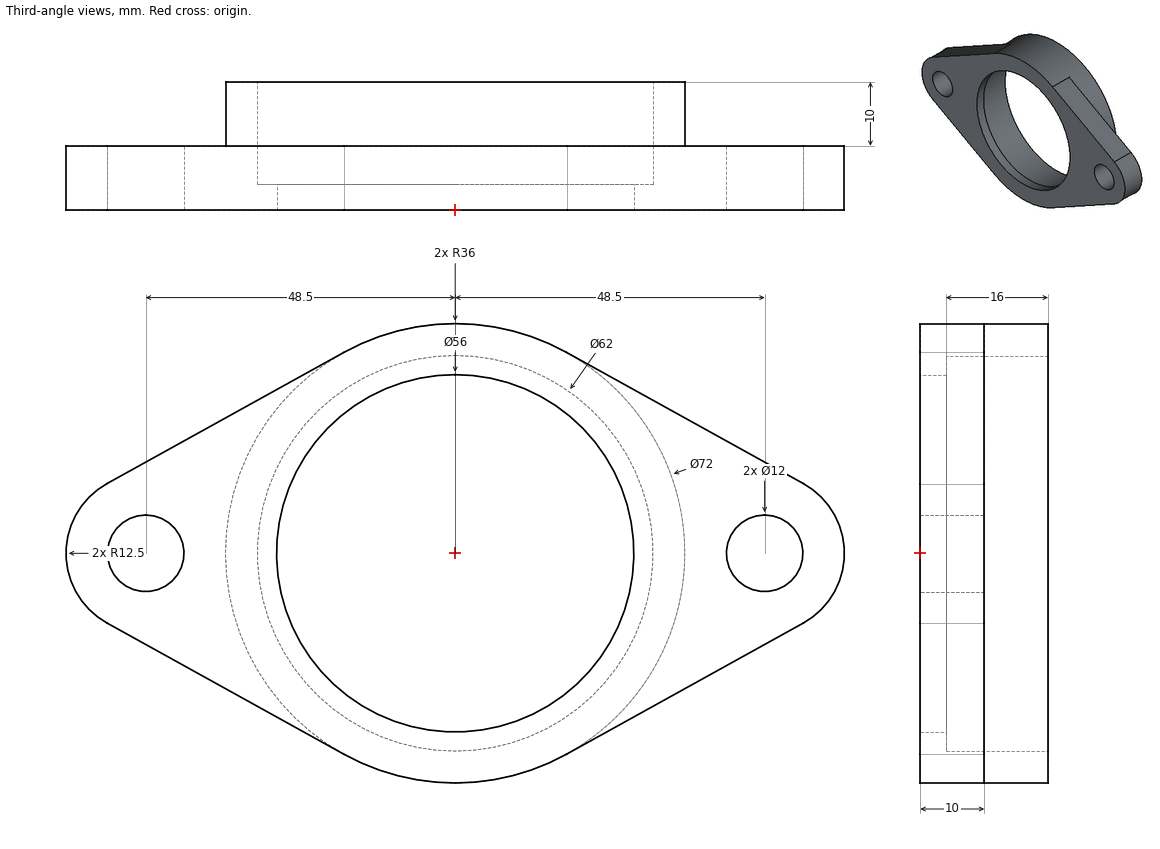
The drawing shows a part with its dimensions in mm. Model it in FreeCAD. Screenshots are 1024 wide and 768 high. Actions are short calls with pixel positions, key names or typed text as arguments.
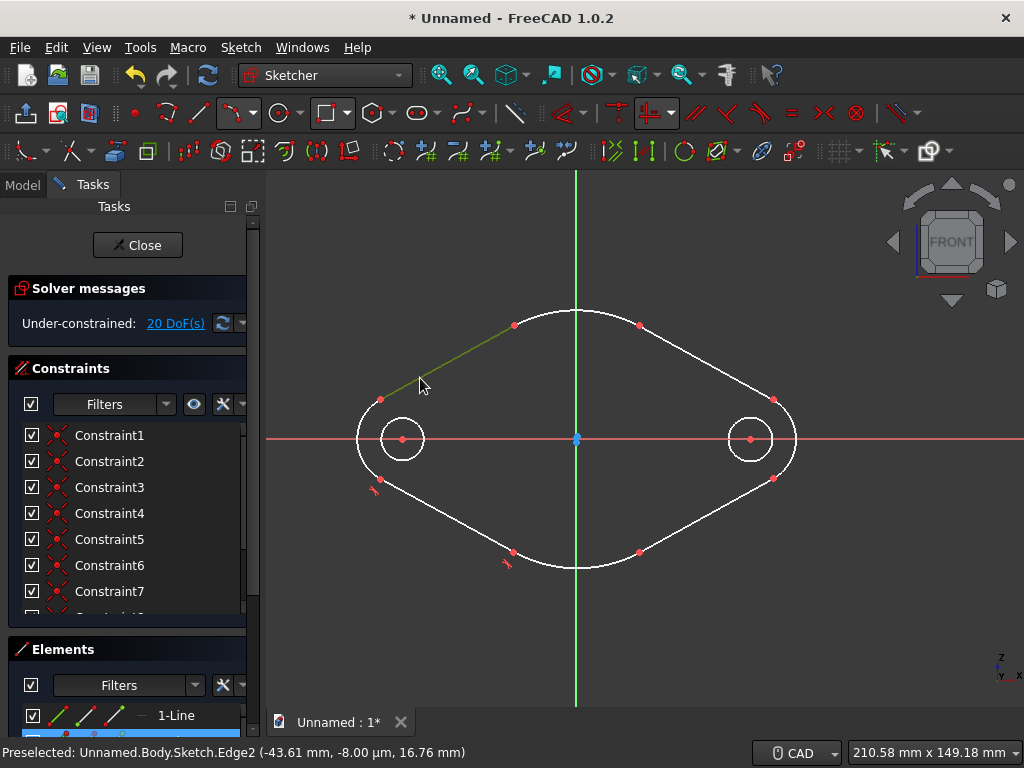
click(361, 421)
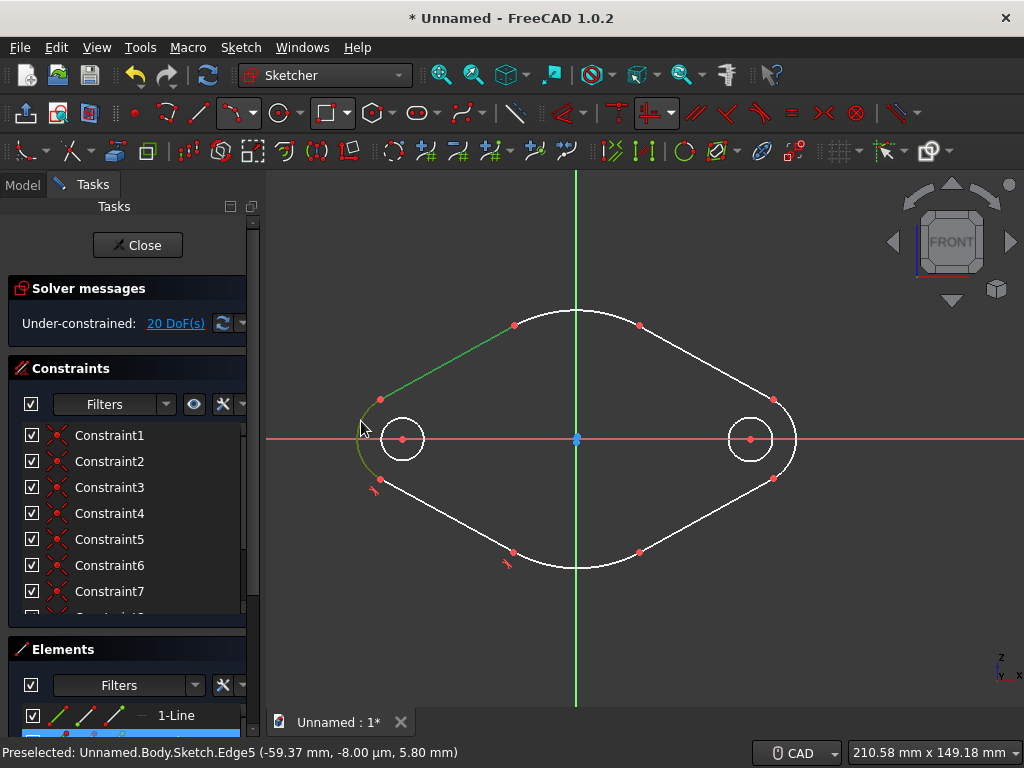
click(760, 114)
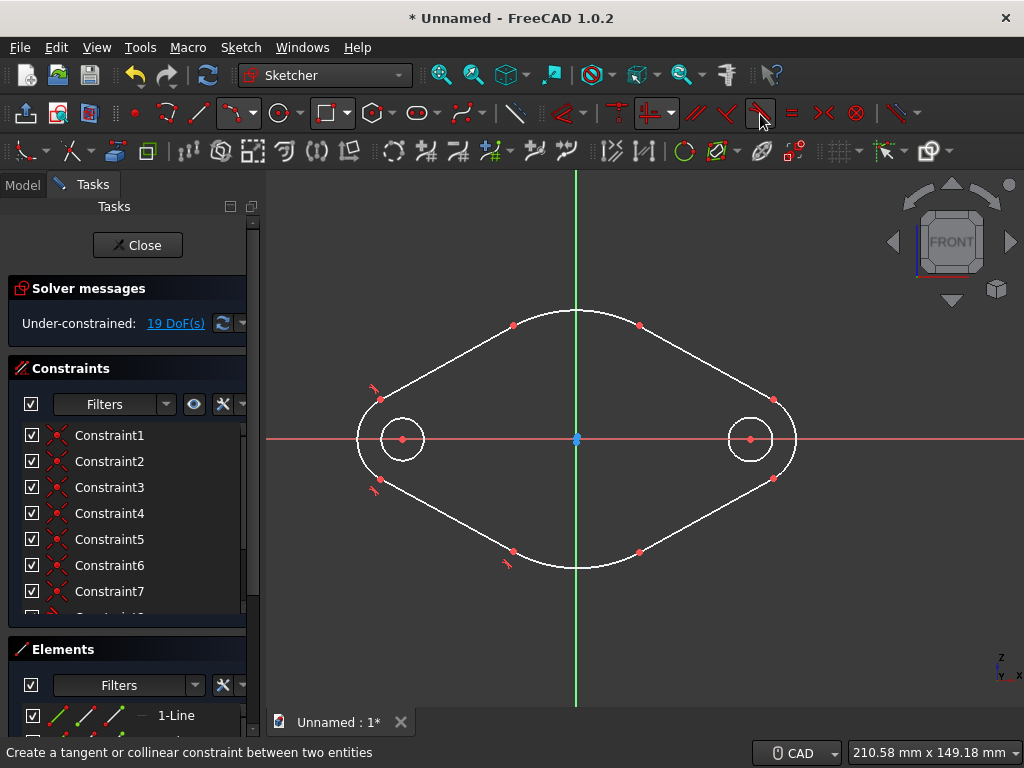
click(421, 378)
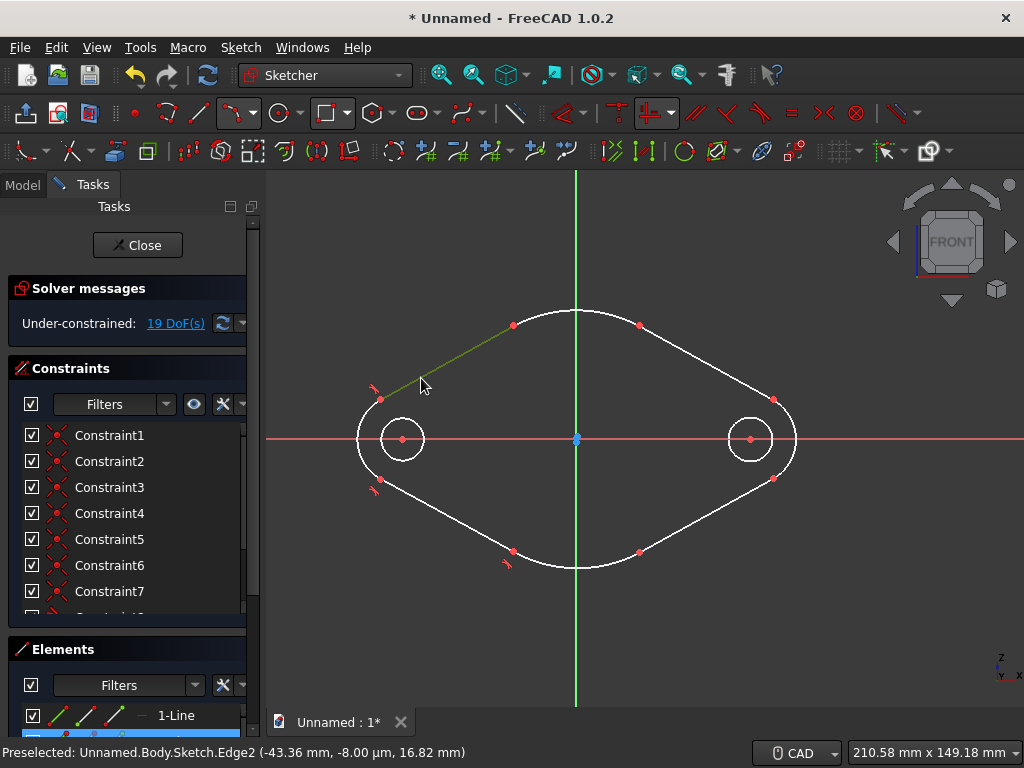
click(602, 313)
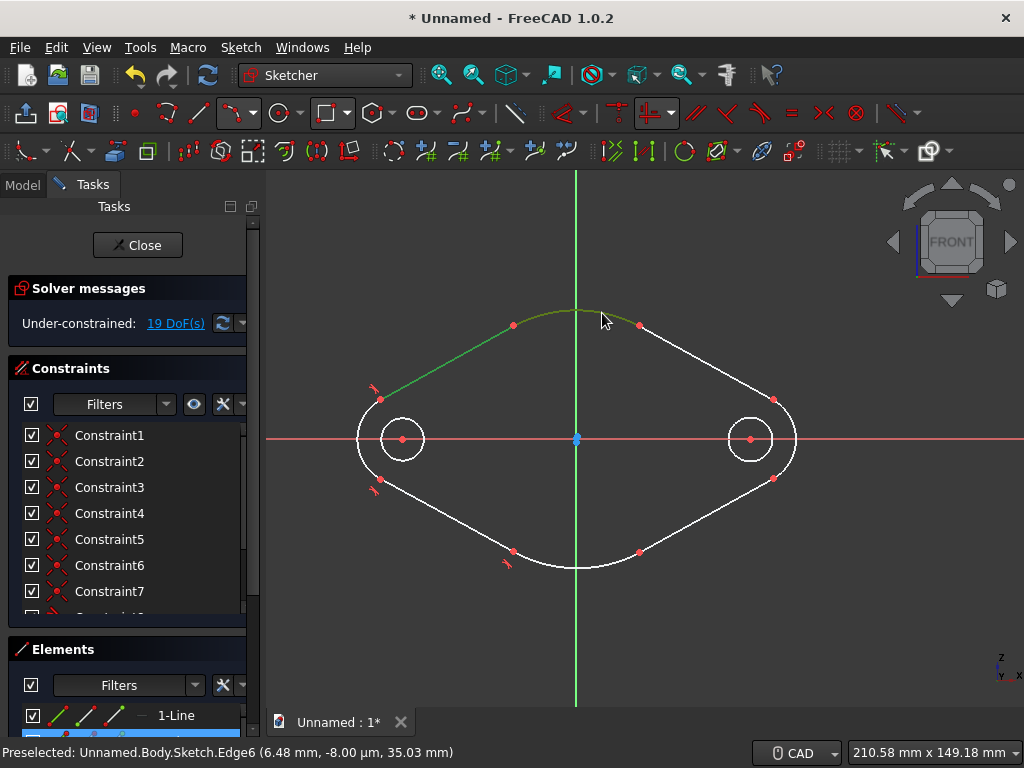
click(760, 114)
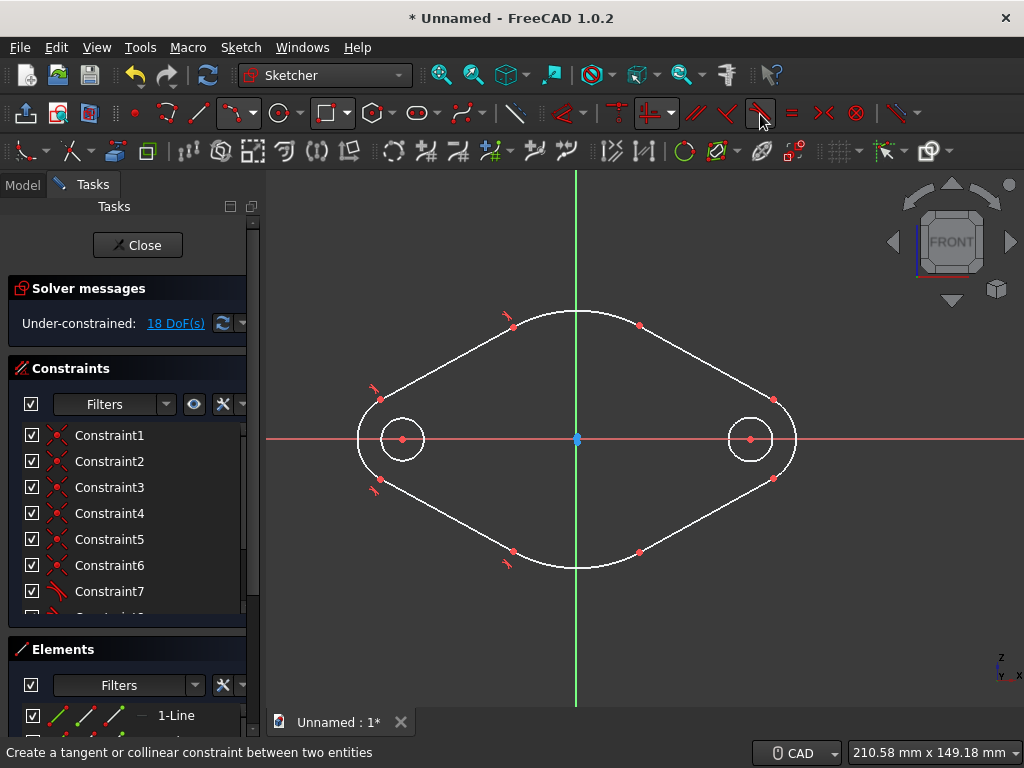
click(679, 348)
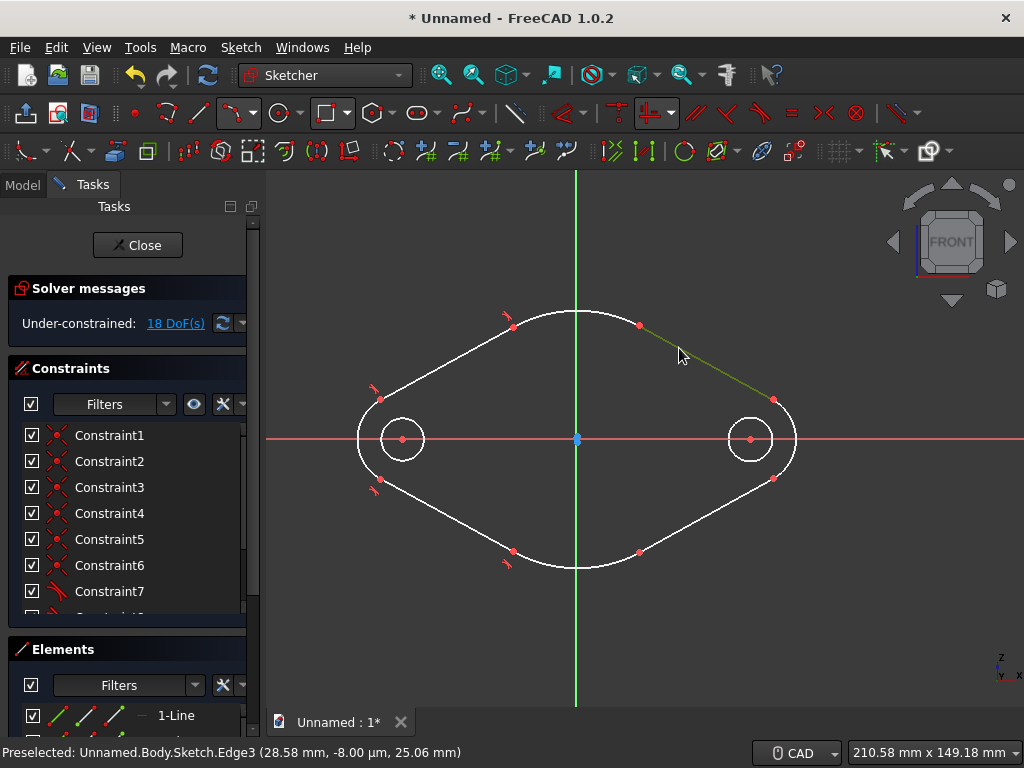
click(602, 313)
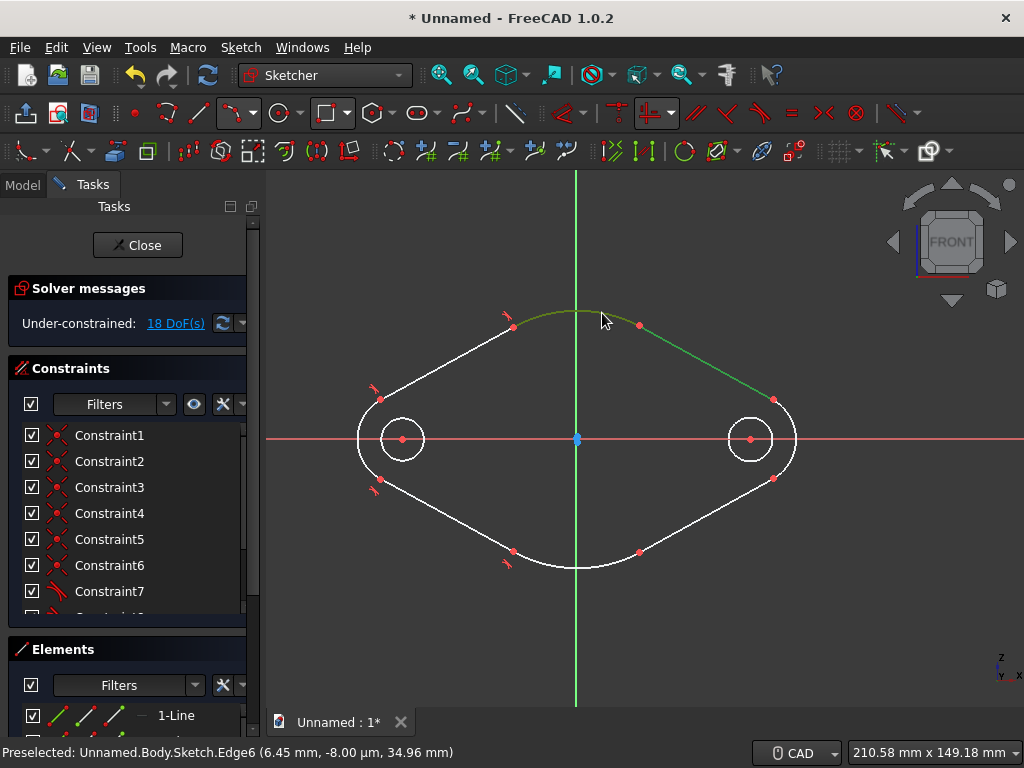
click(760, 114)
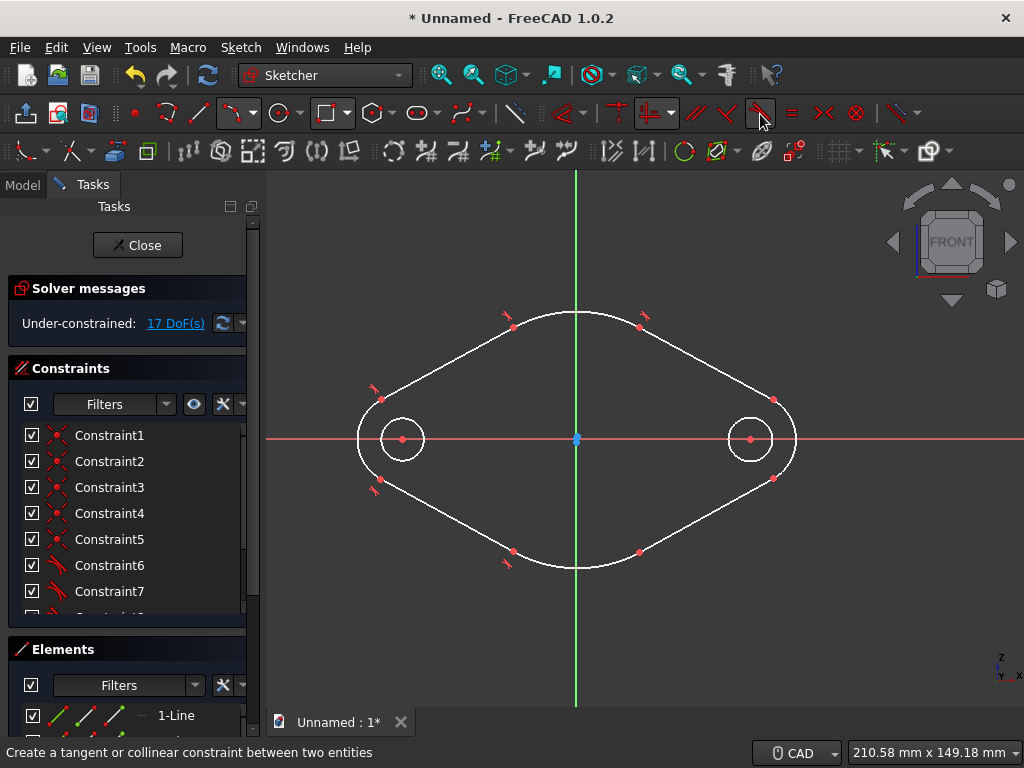
click(679, 349)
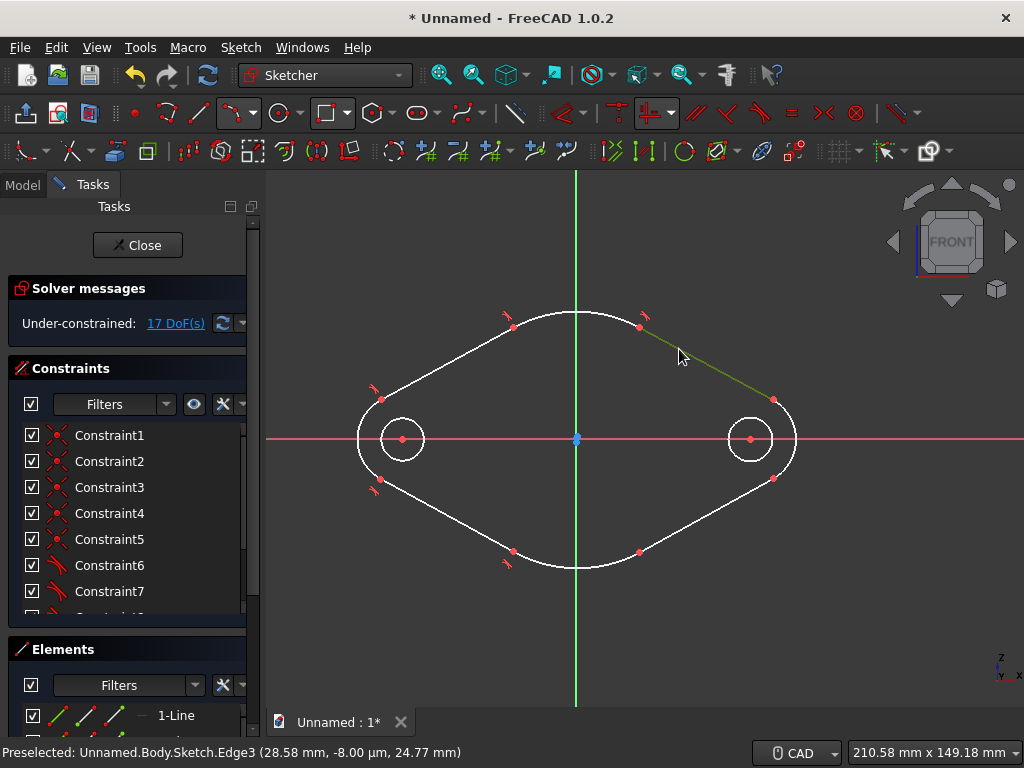
click(792, 458)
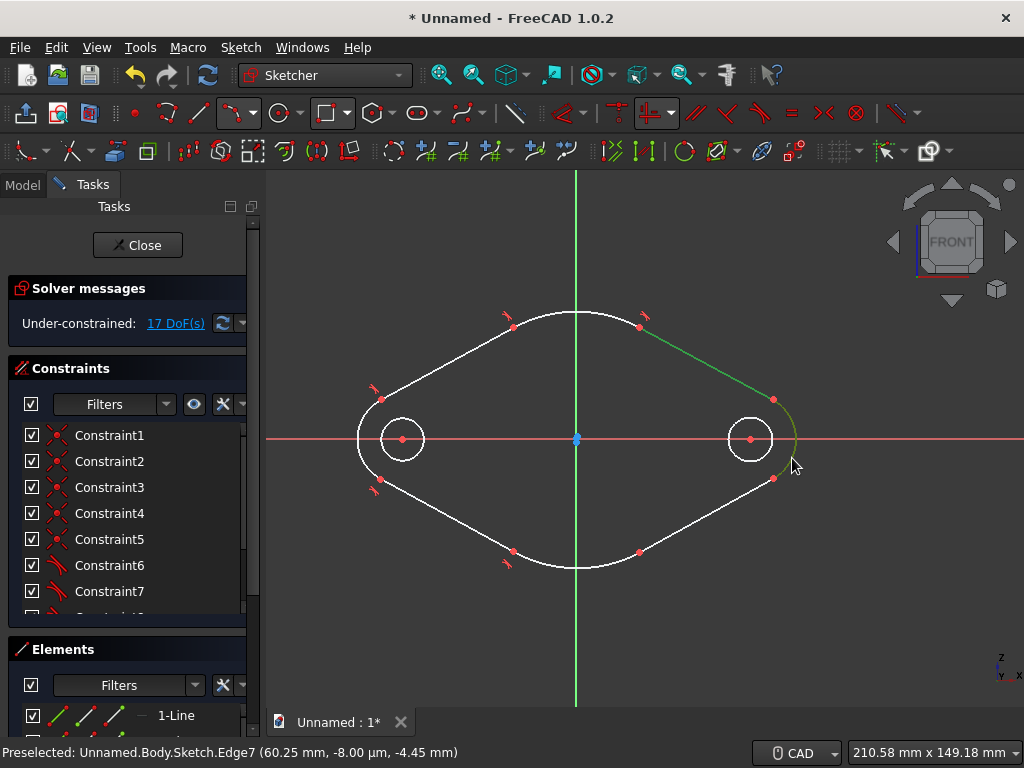
click(760, 114)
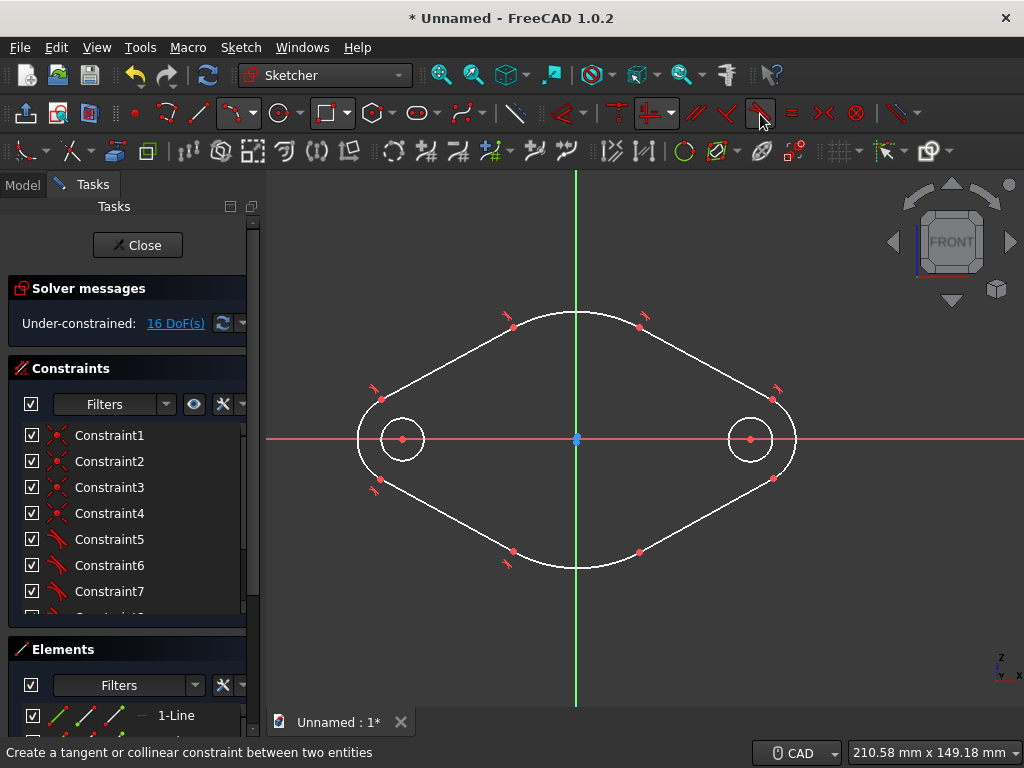
click(733, 501)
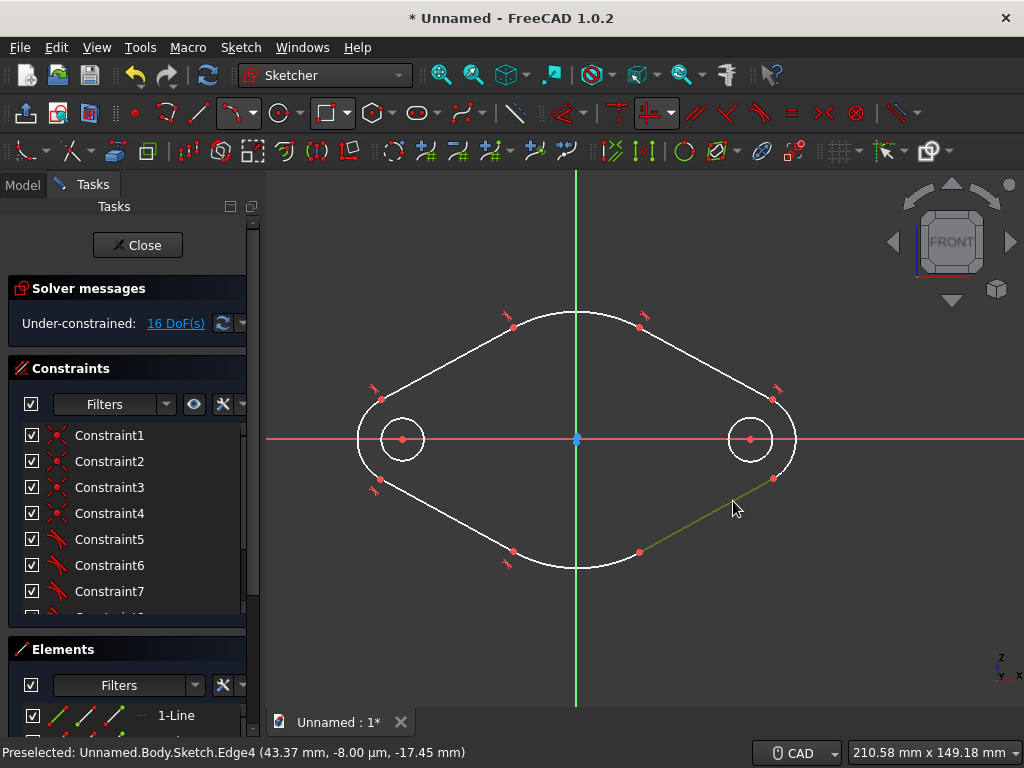
click(792, 458)